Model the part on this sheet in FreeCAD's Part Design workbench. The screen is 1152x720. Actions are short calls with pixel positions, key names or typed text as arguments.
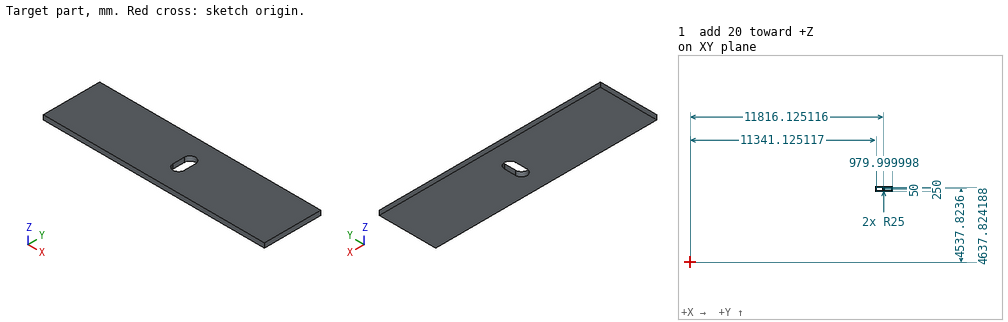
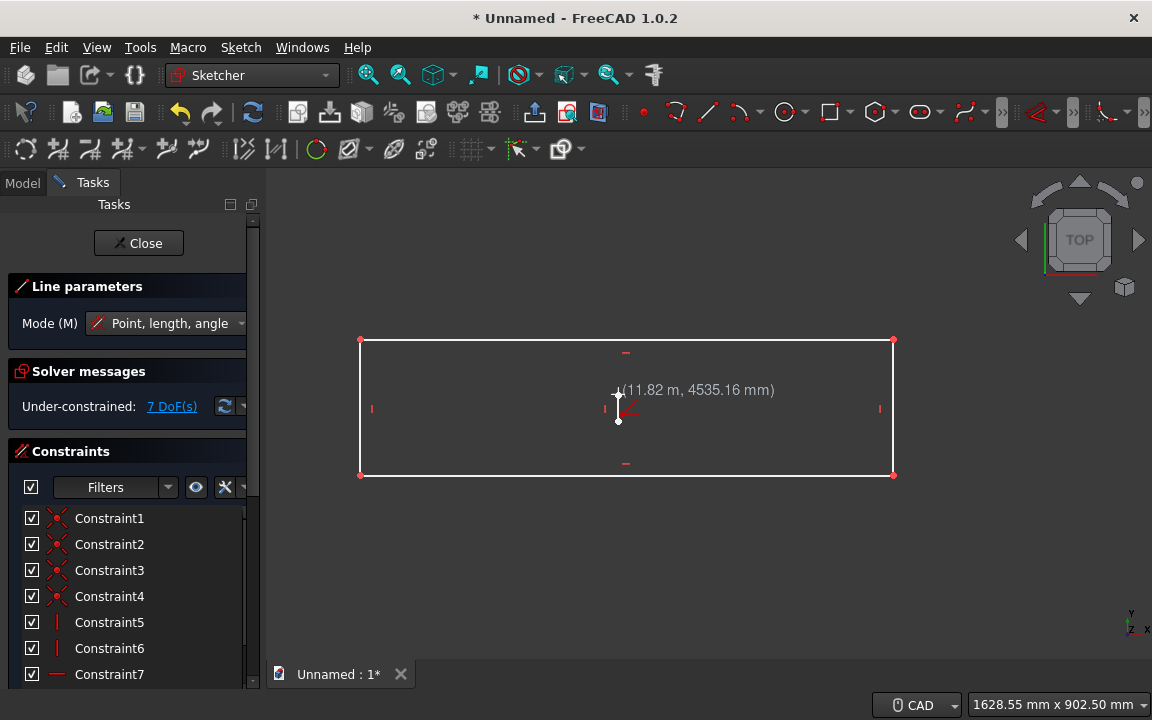
click(646, 394)
click(646, 421)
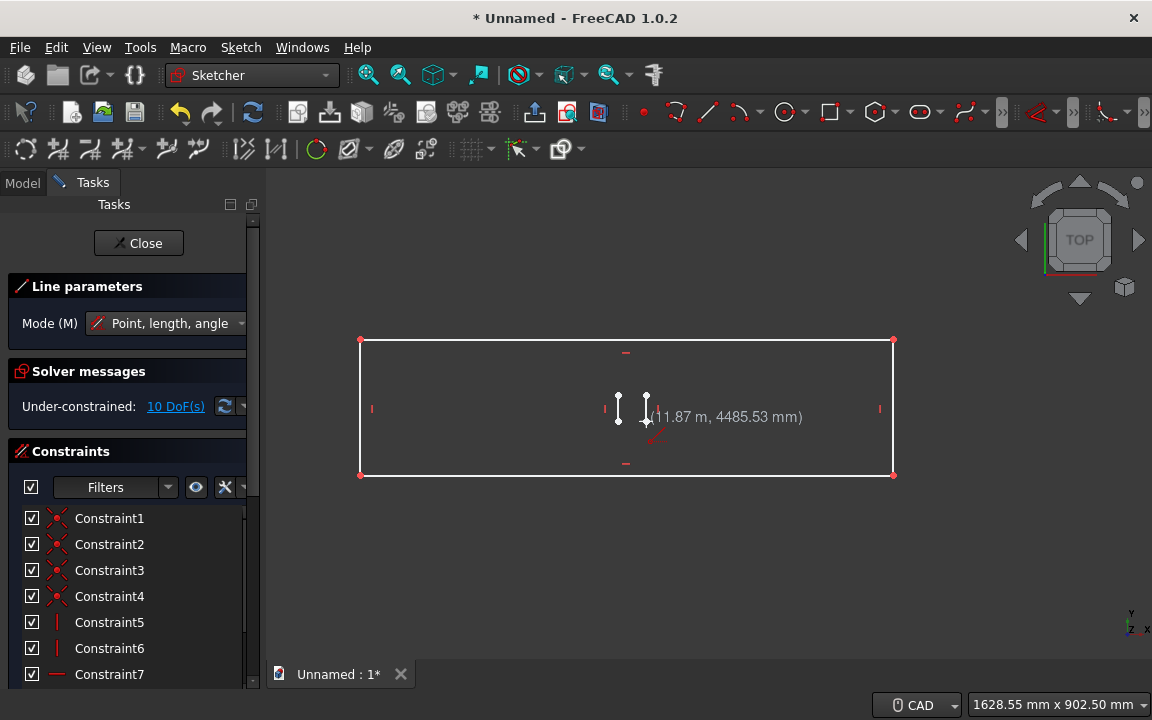
key(g)
key(3)
key(a)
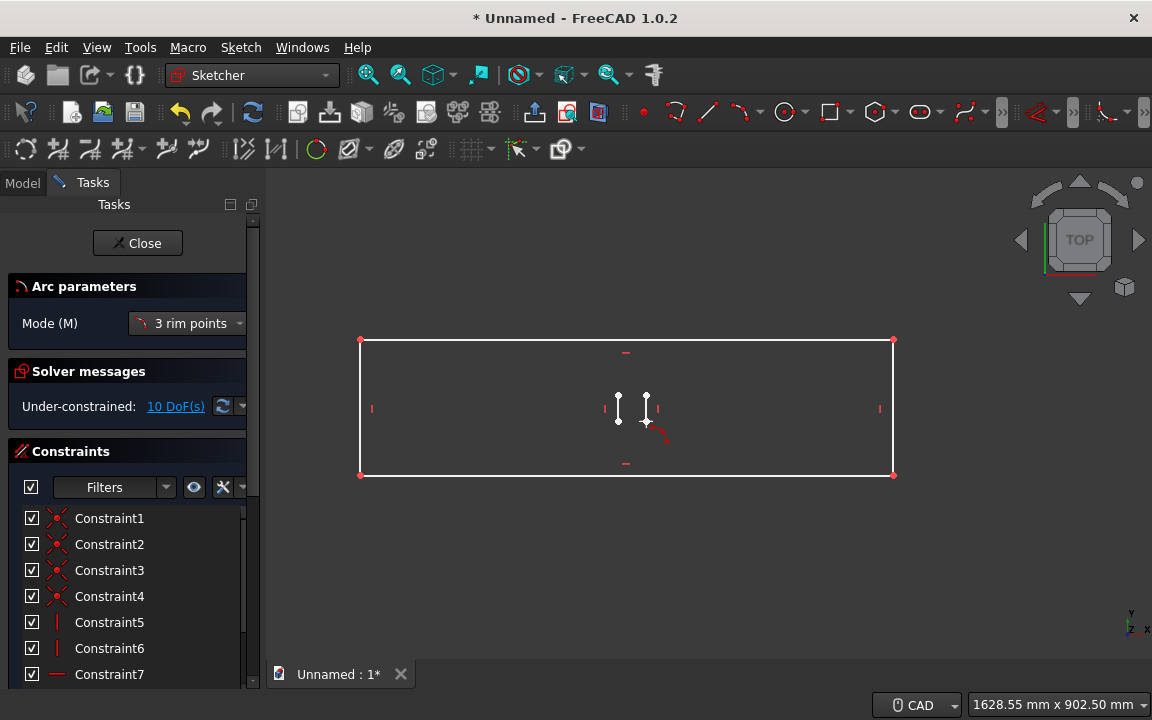
click(618, 395)
click(646, 395)
click(632, 380)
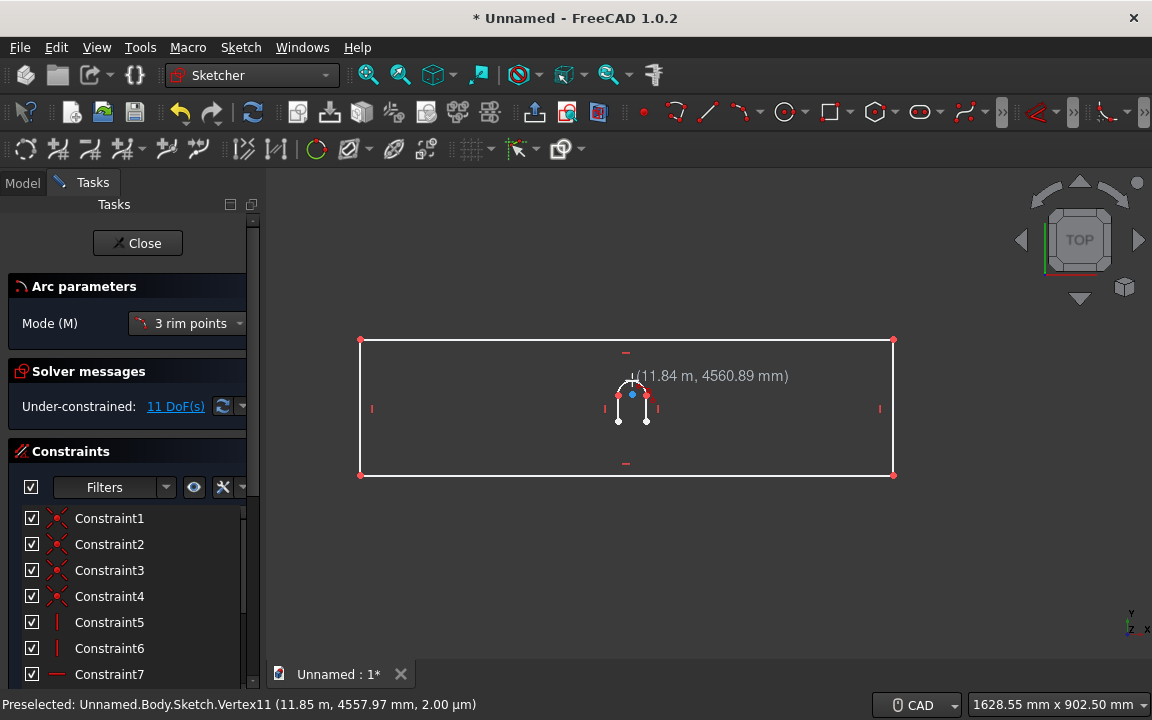
click(646, 422)
click(618, 422)
click(632, 434)
key(Escape)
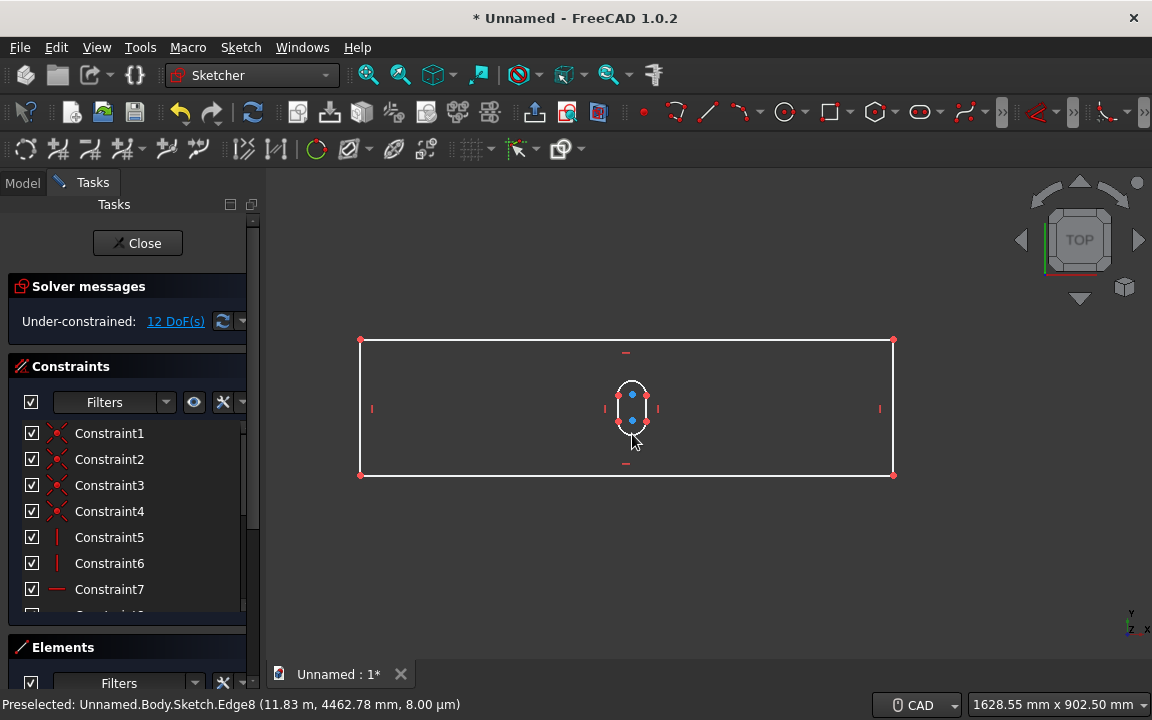
scroll(618, 411, up, 2)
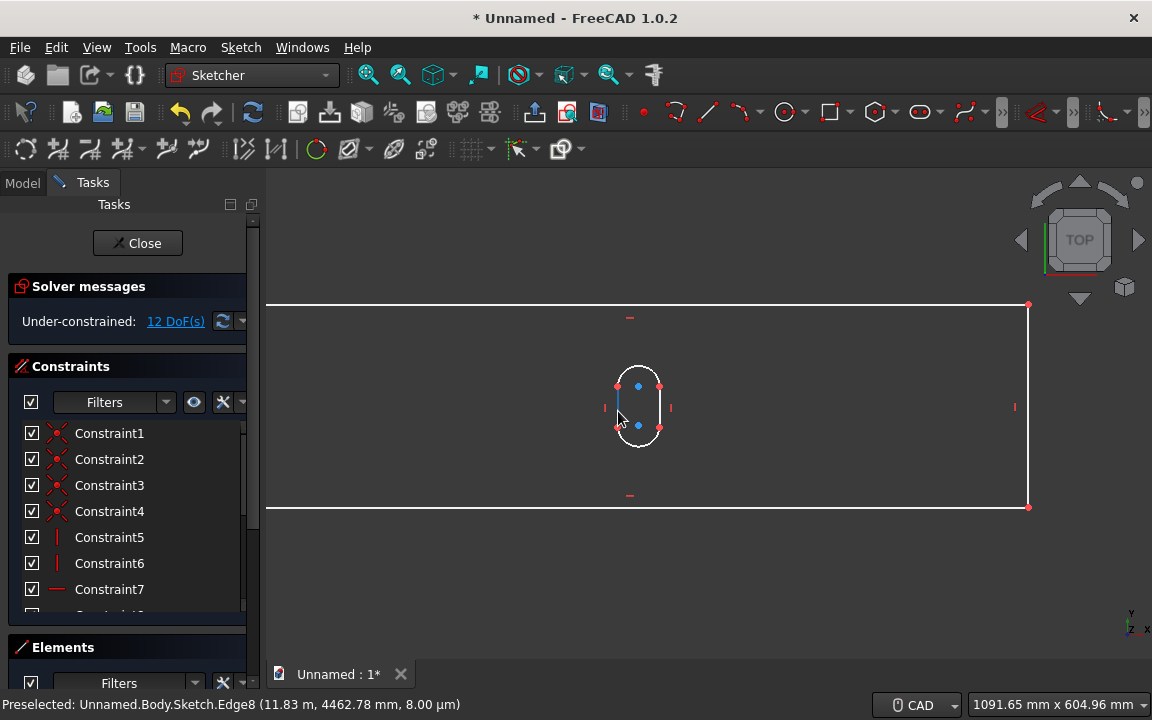
click(618, 411)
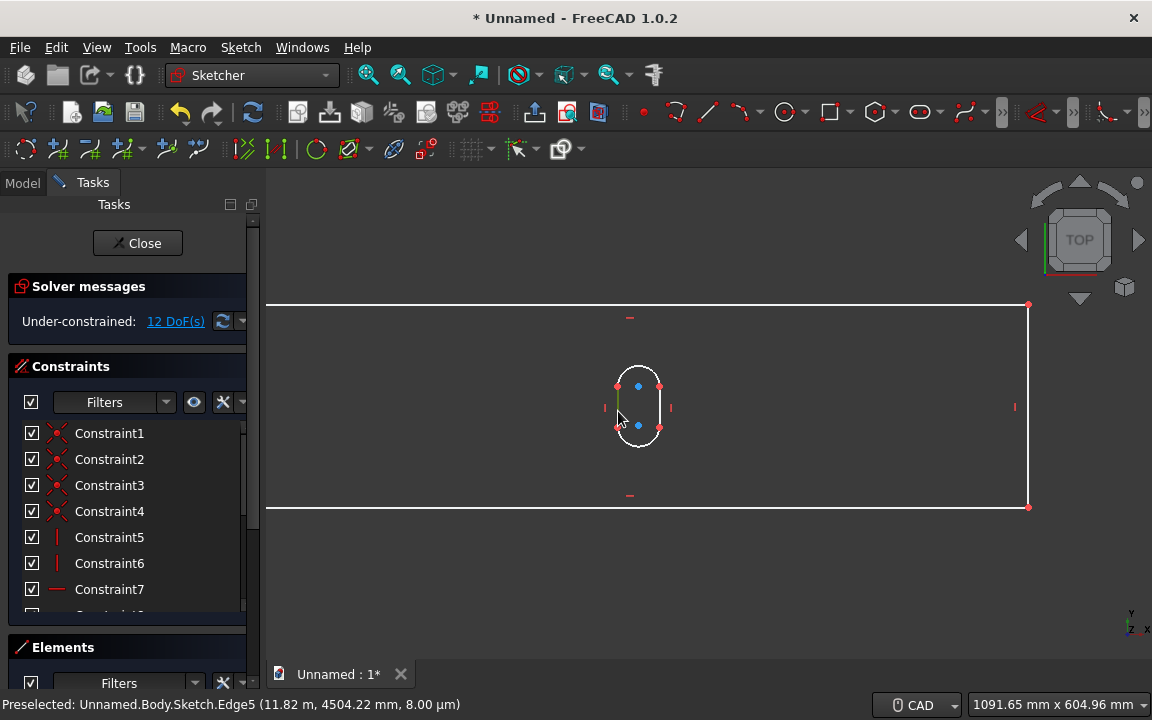
click(651, 370)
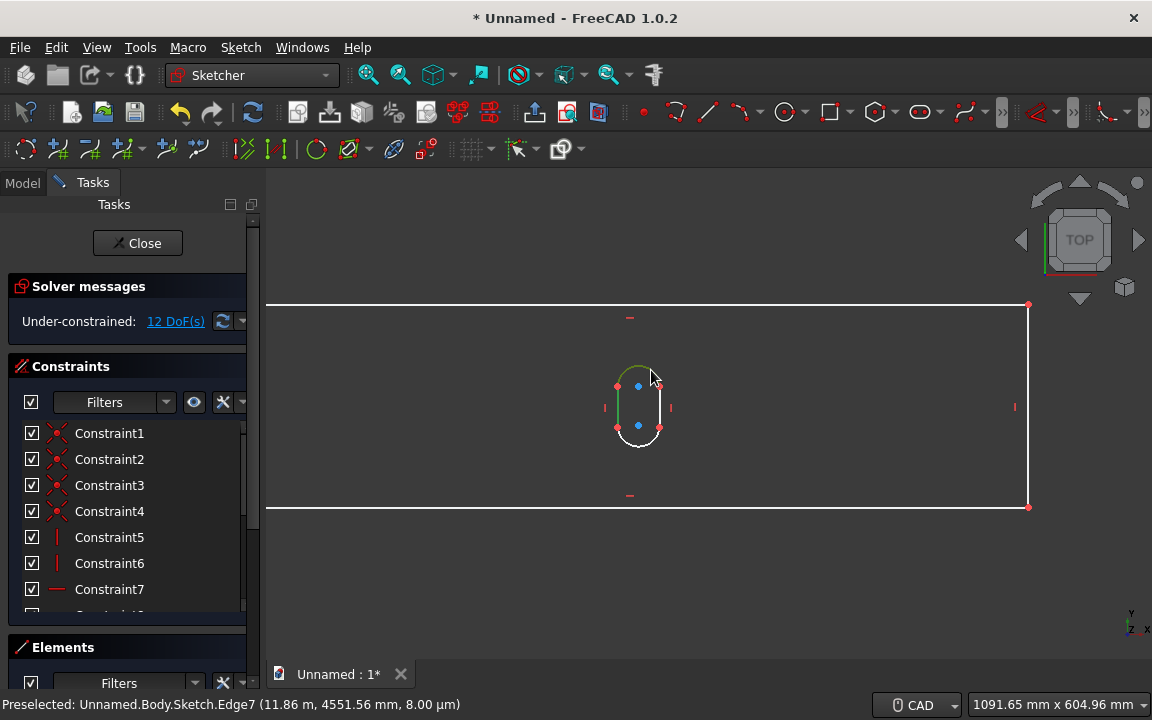
key(t)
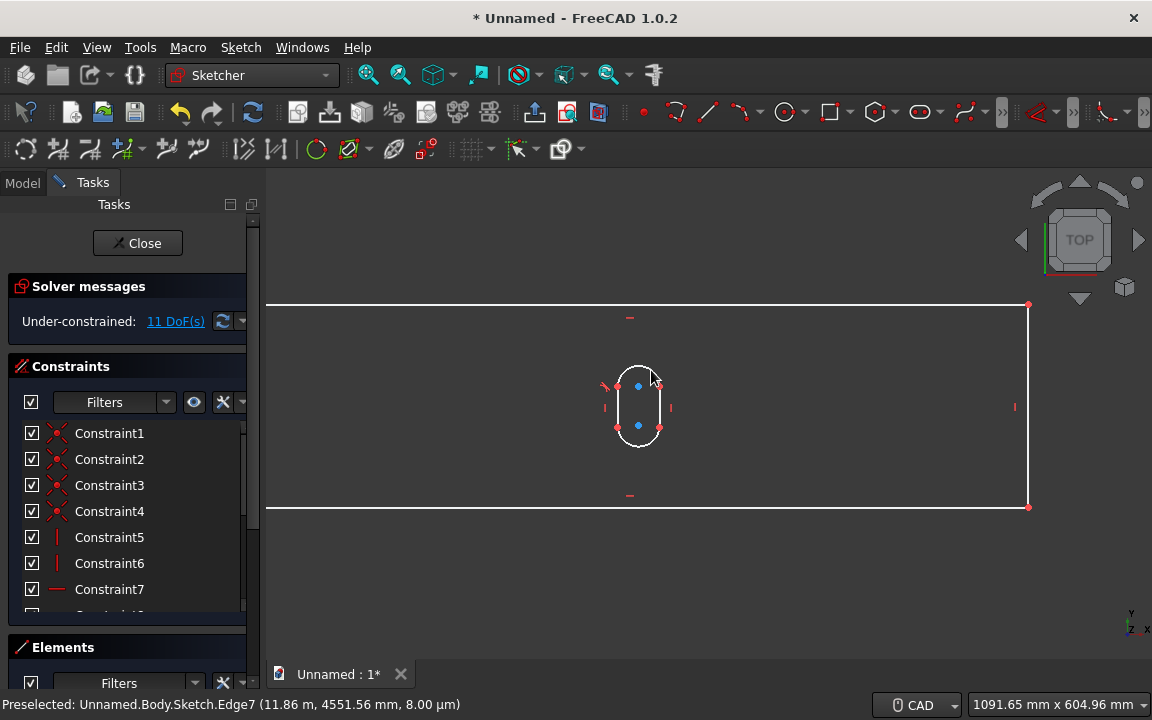
click(618, 415)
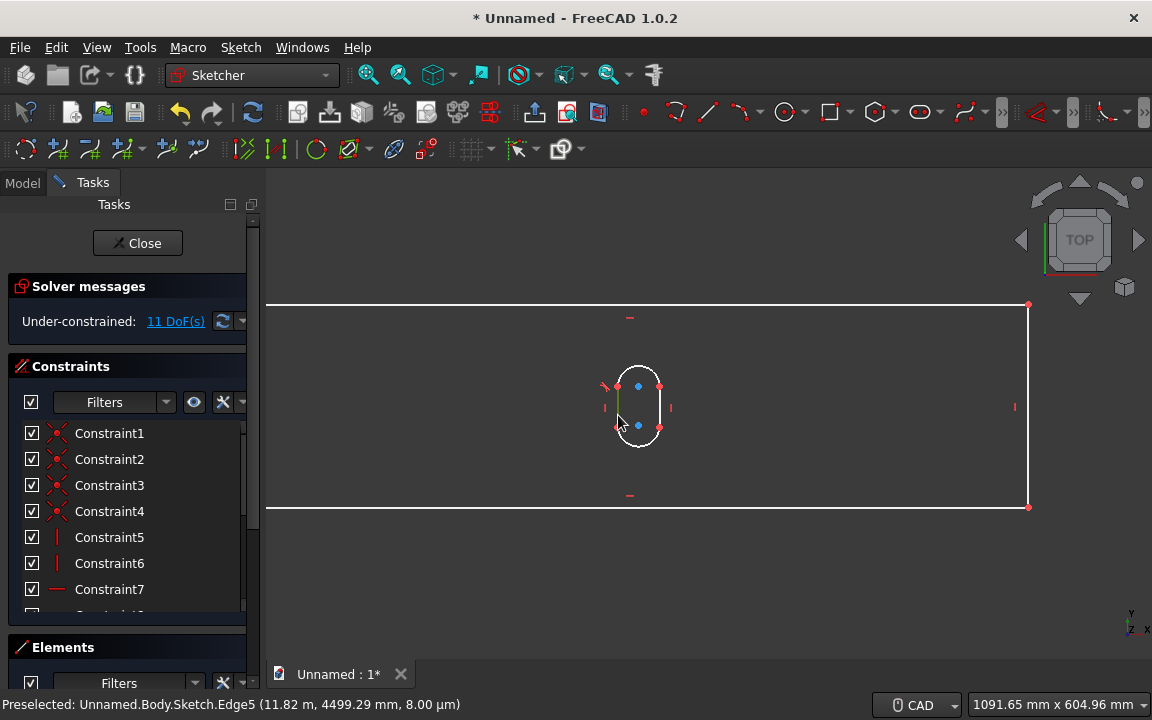
click(627, 443)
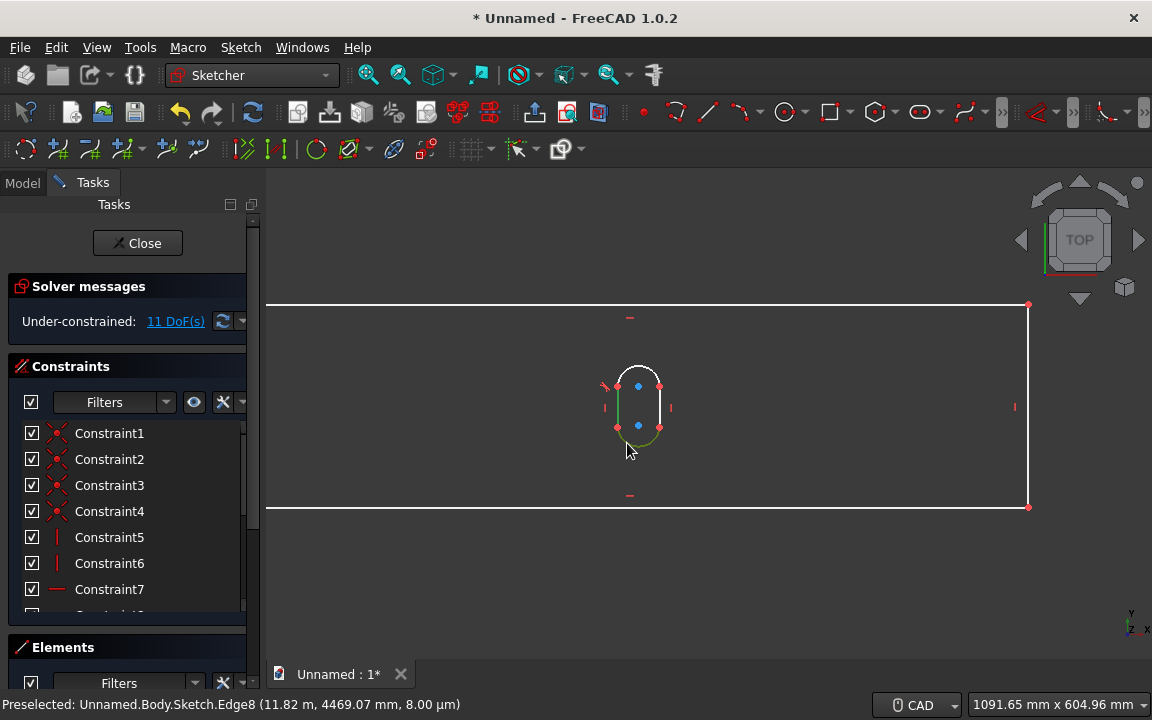
key(t)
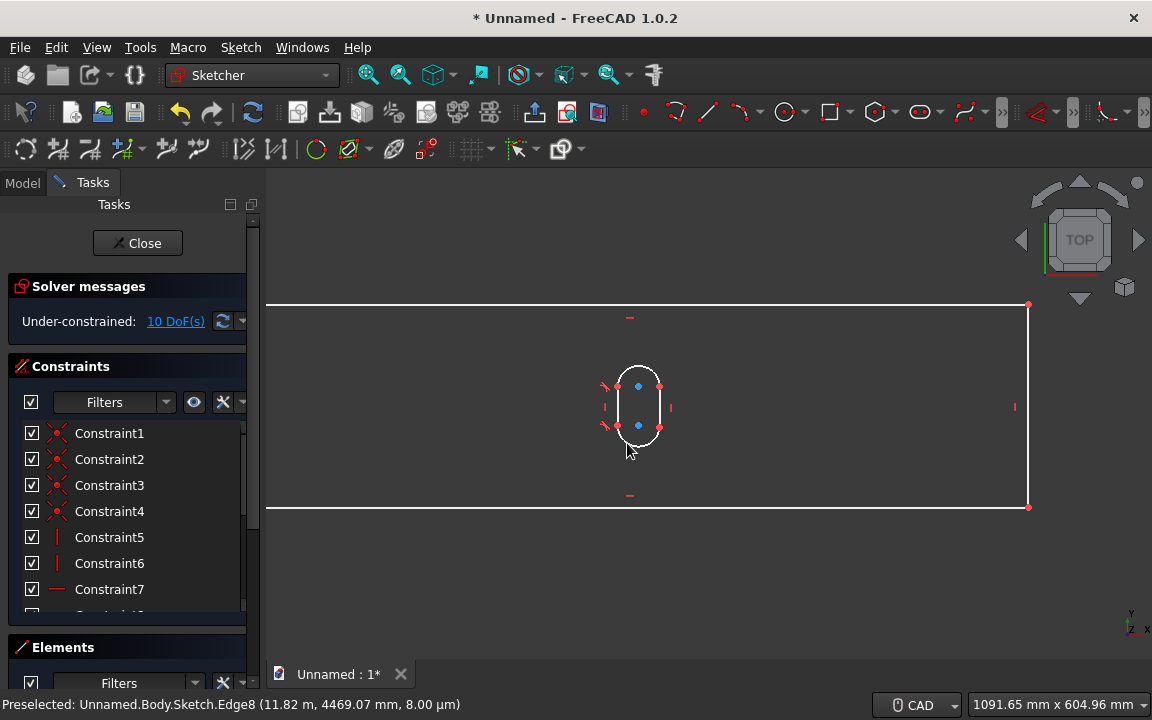
click(660, 399)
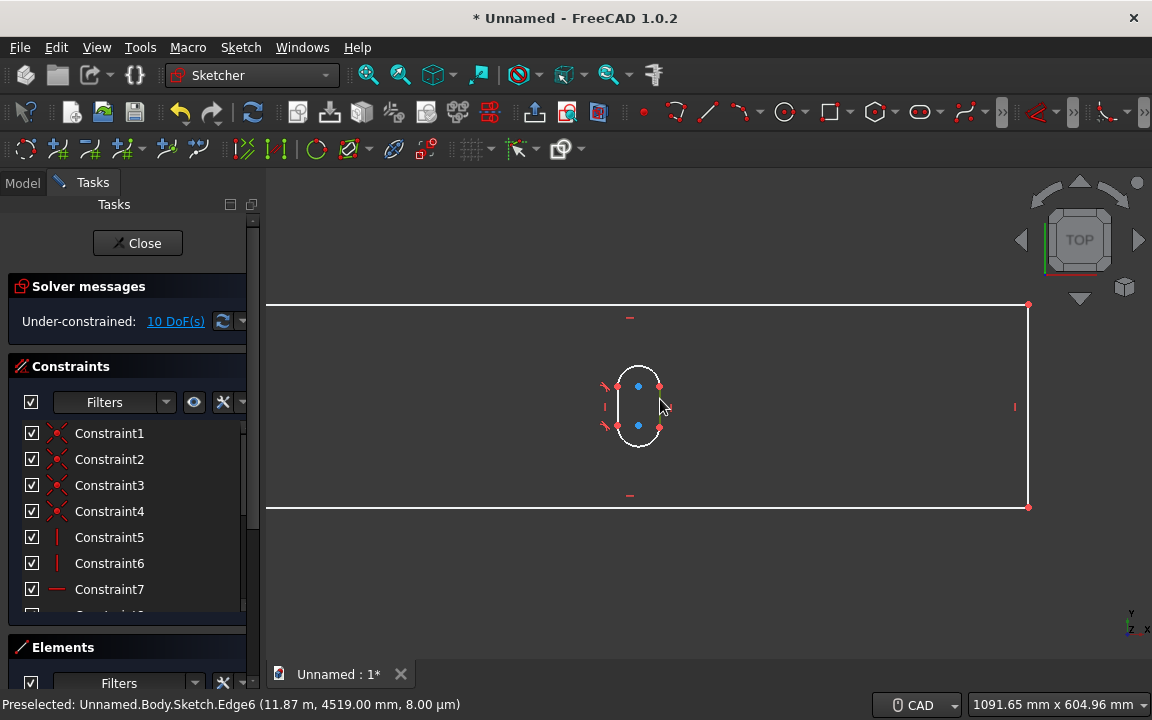
click(651, 370)